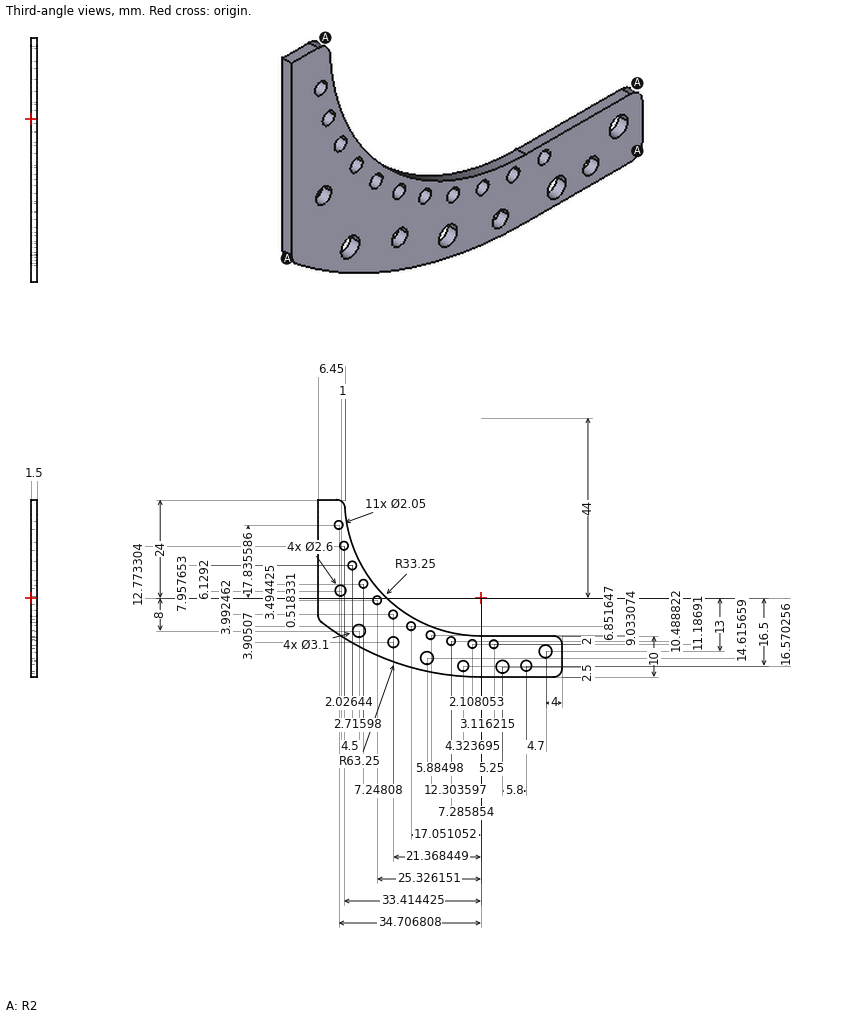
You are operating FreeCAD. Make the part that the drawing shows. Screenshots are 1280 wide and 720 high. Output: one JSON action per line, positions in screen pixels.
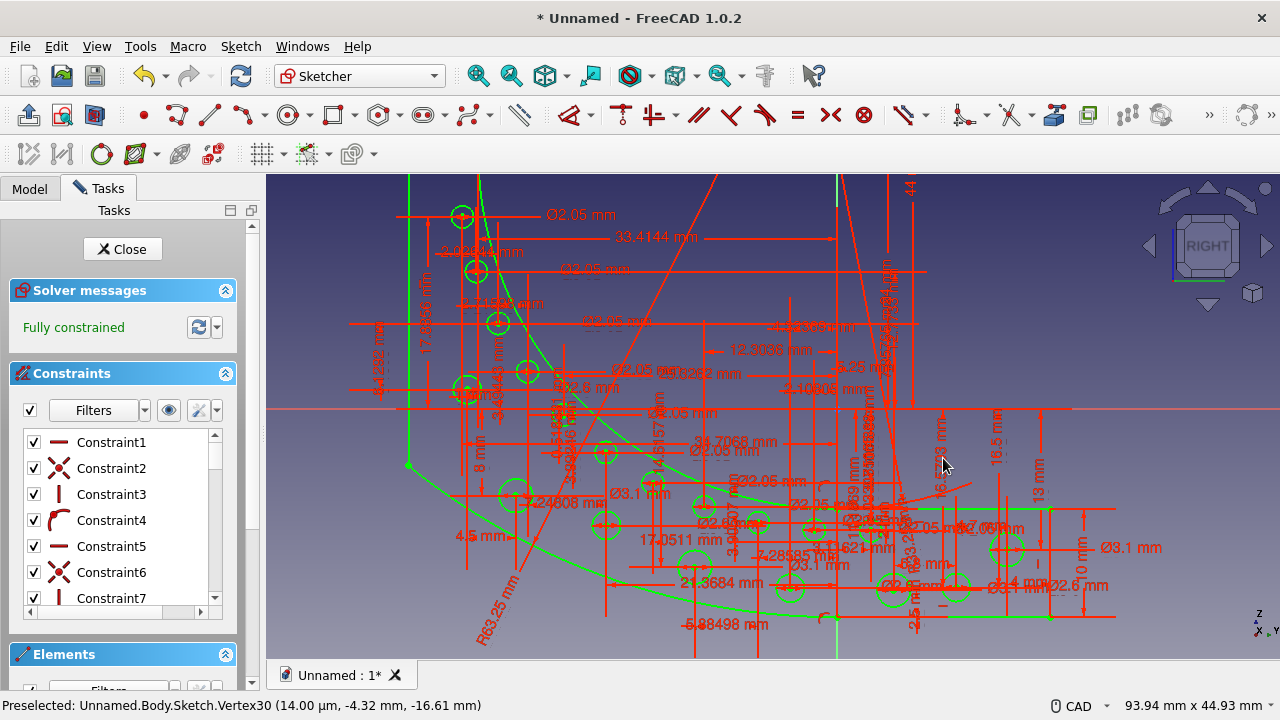
{"action": "left_click", "coordinate": [123, 249]}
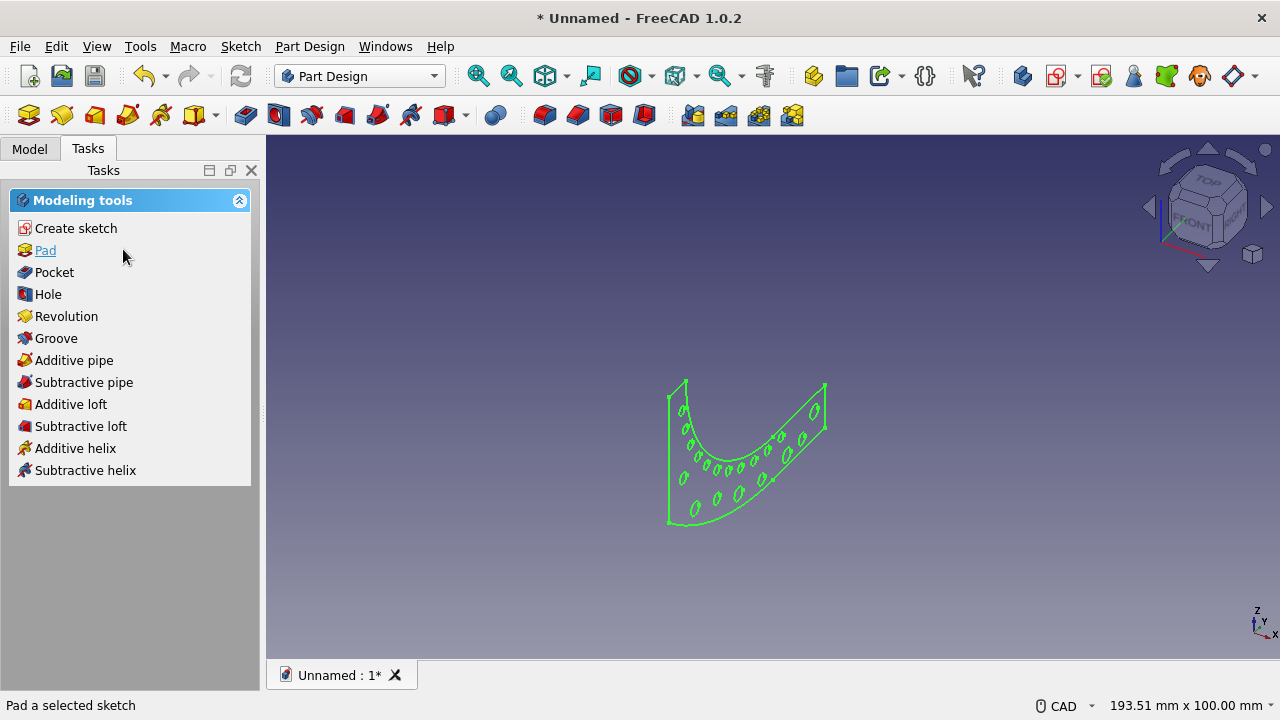
{"action": "left_click", "coordinate": [29, 116]}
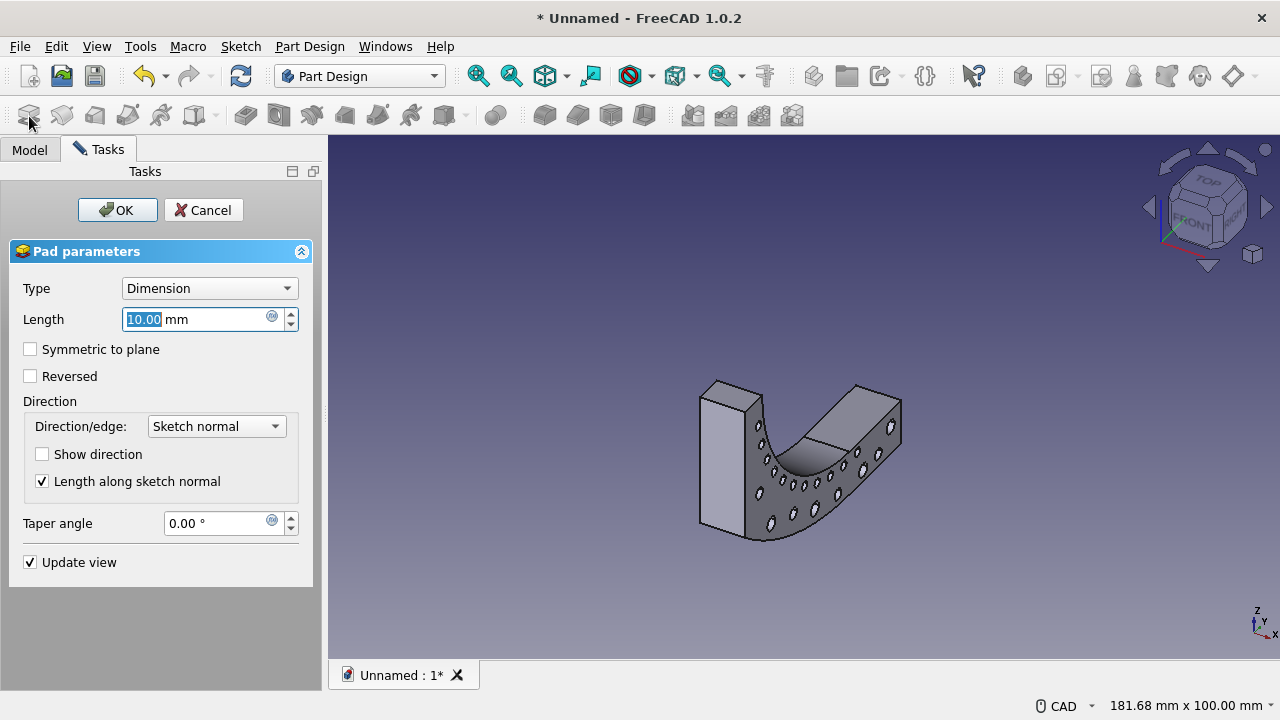
{"action": "type", "text": "1.5"}
{"action": "key", "text": "Tab"}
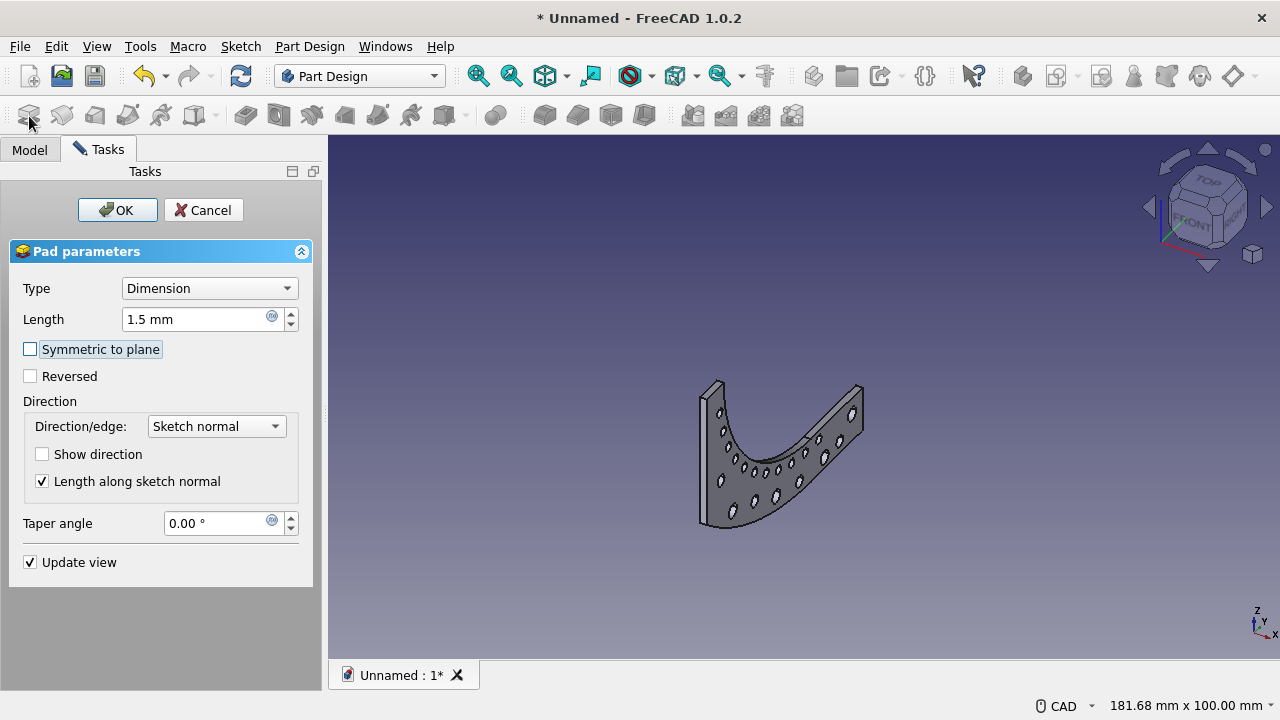
{"action": "left_click", "coordinate": [118, 210]}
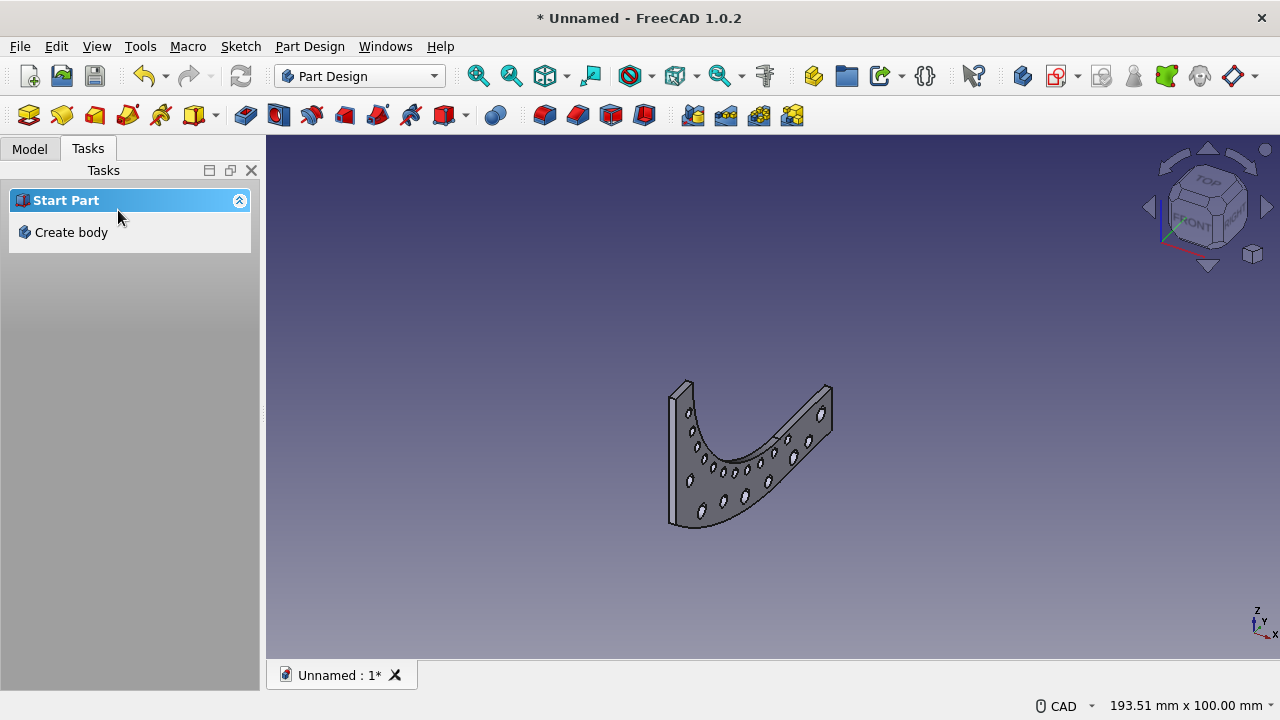
{"action": "scroll", "coordinate": [828, 428], "scroll_direction": "up", "scroll_amount": 9}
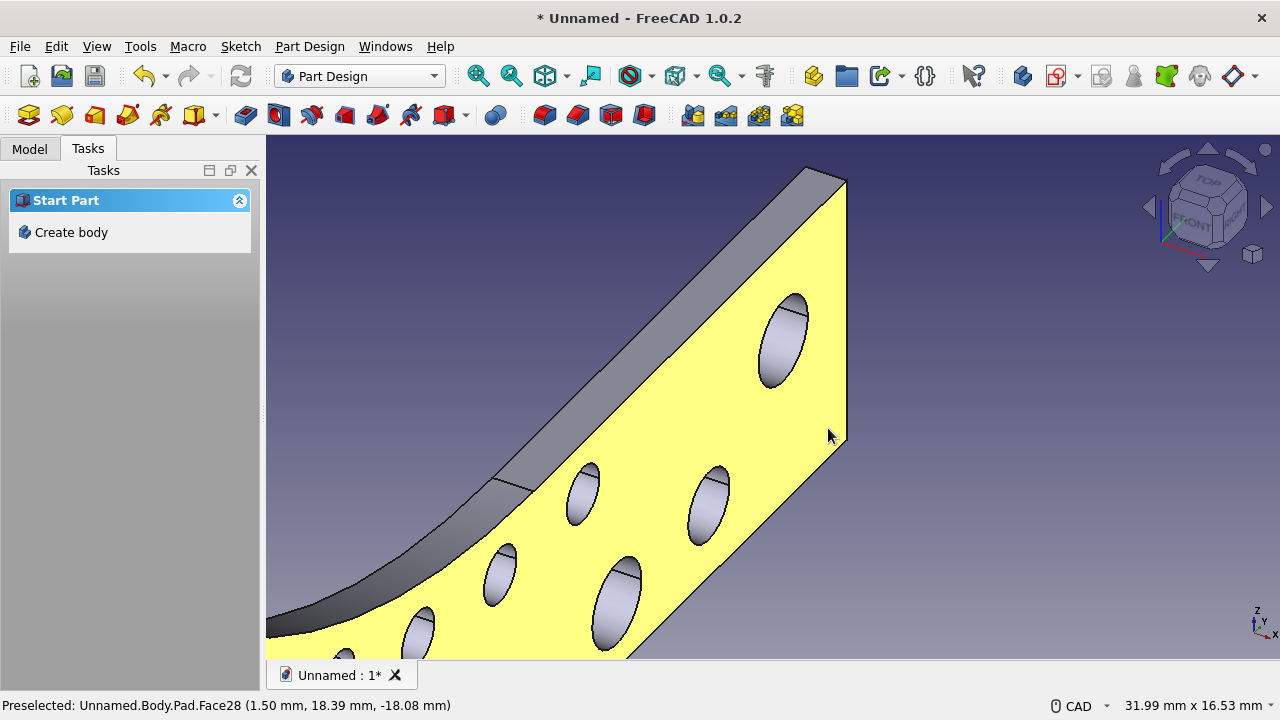
{"action": "left_click", "coordinate": [479, 76]}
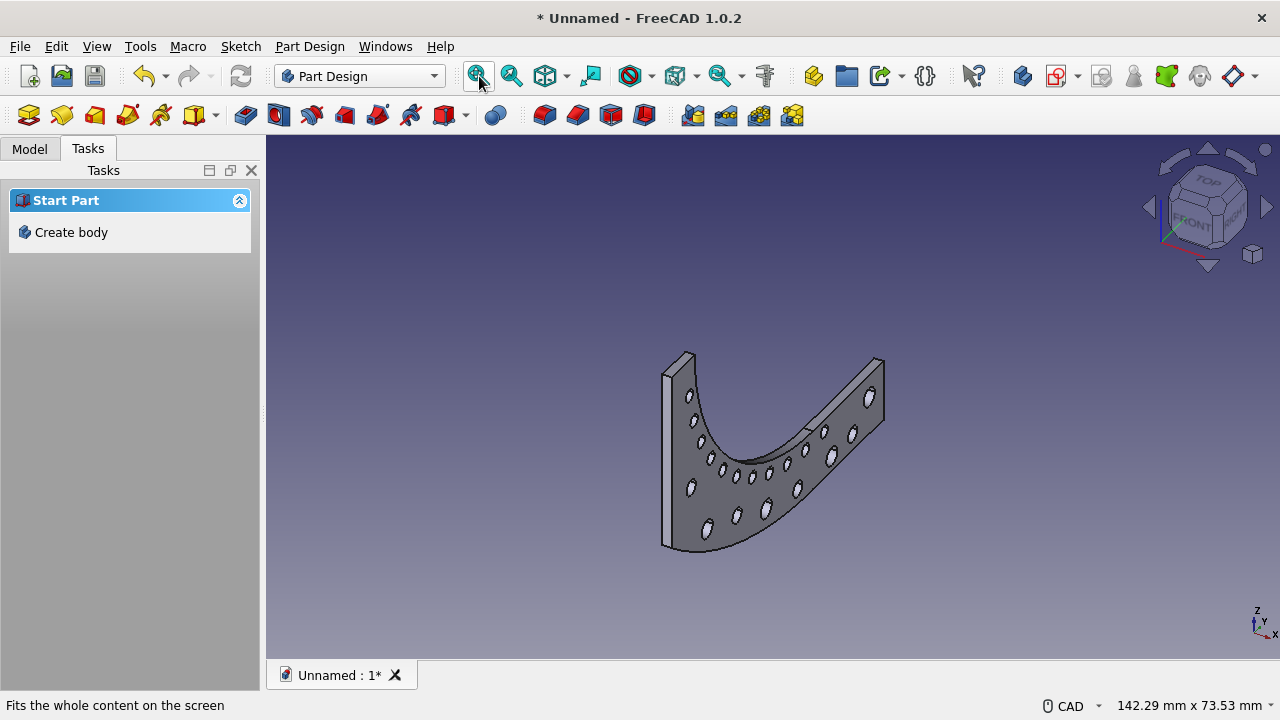
{"action": "key", "text": "0"}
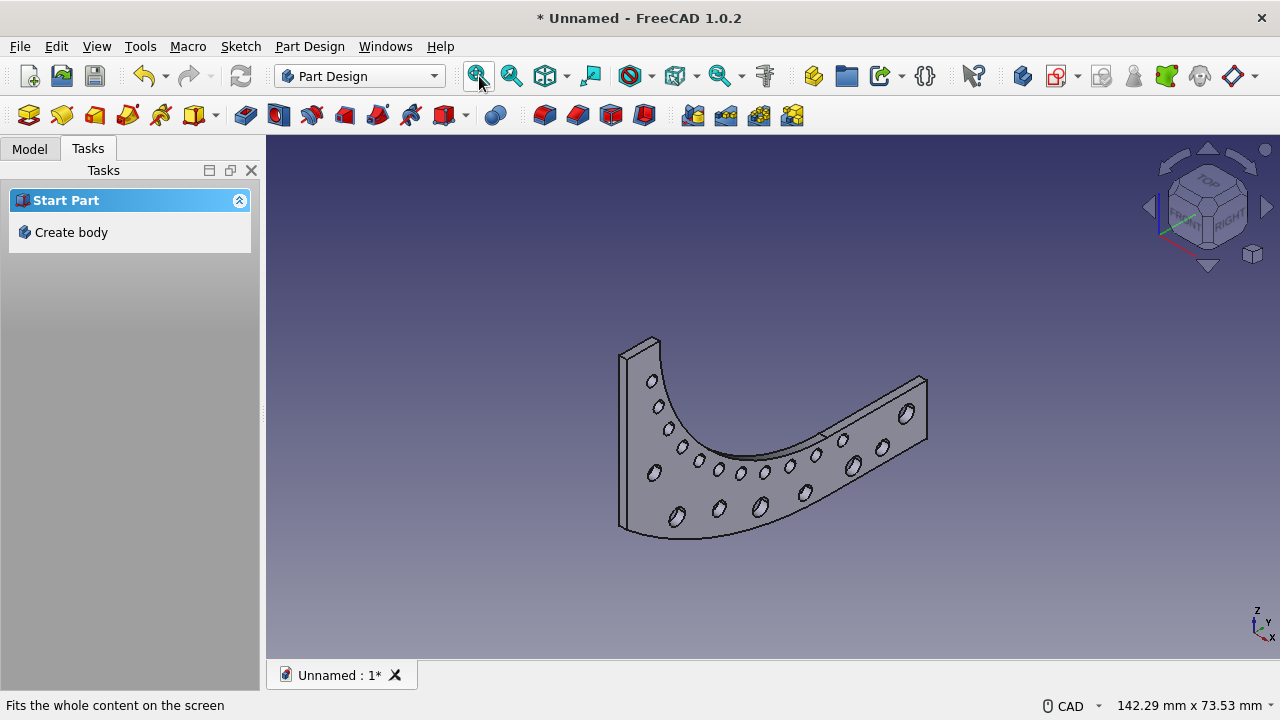
{"action": "scroll", "coordinate": [923, 435], "scroll_direction": "up", "scroll_amount": 7}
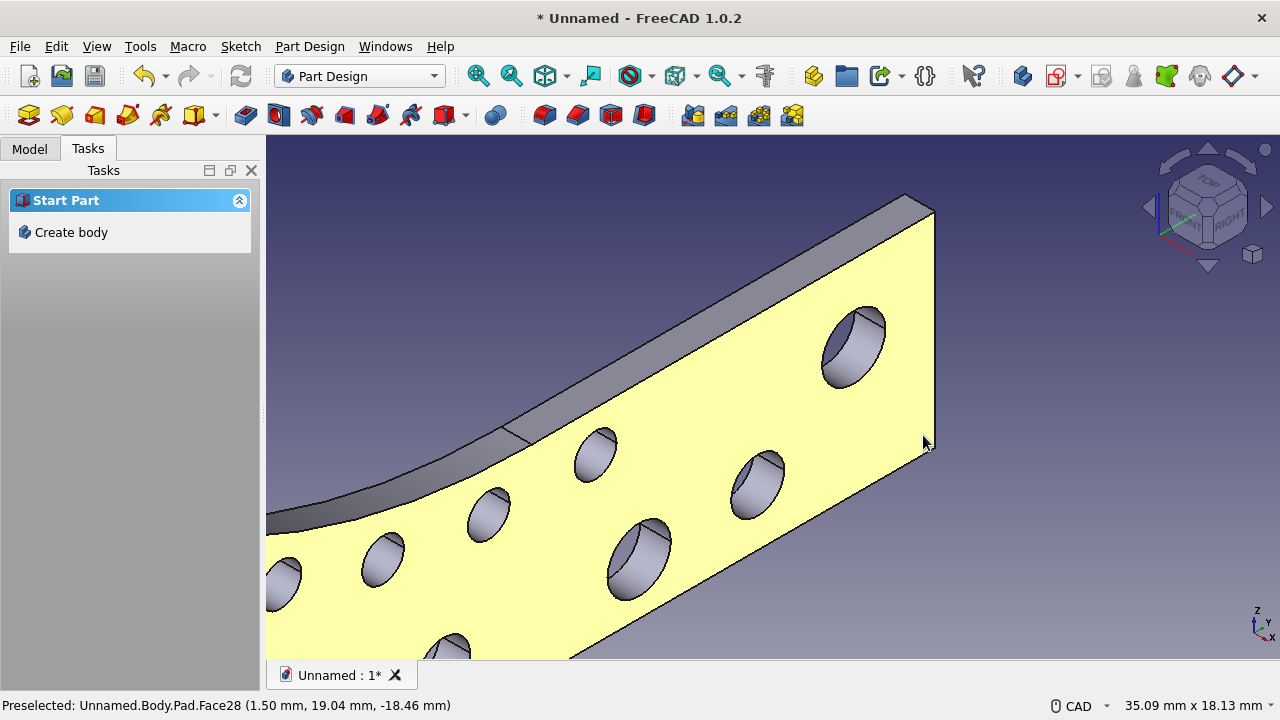
{"action": "key", "text": "v f"}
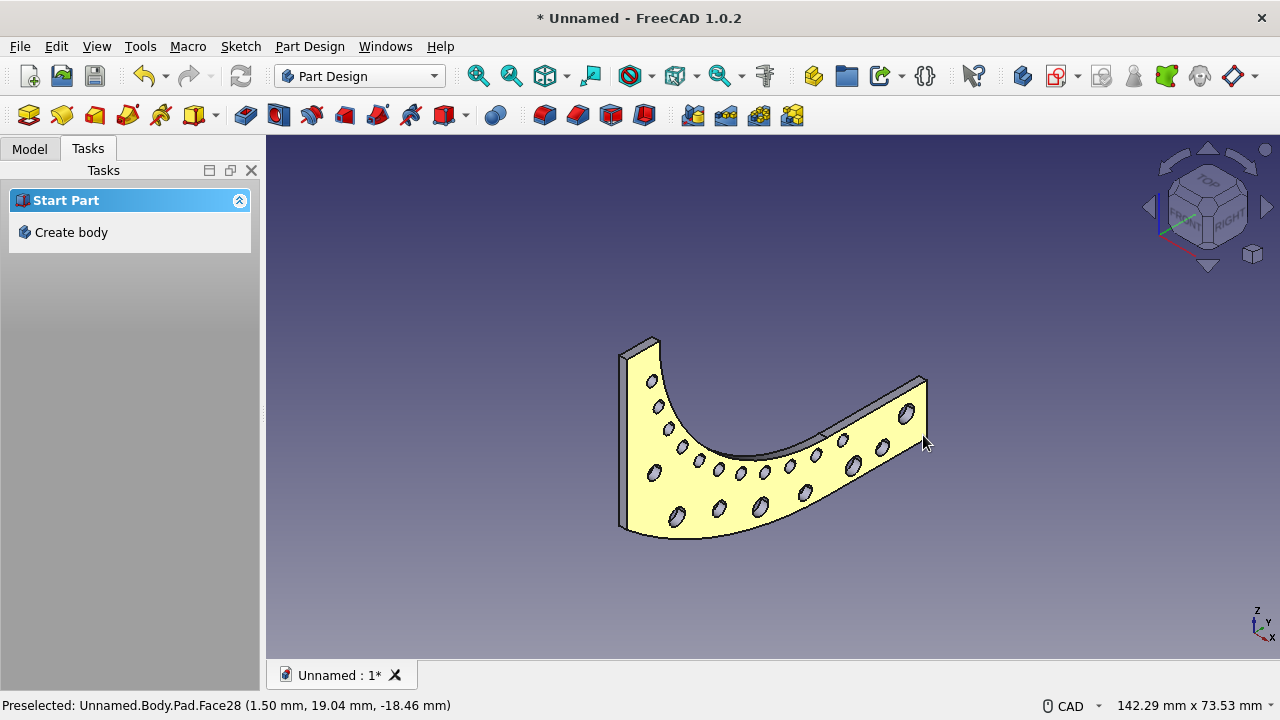
{"action": "key", "text": "2"}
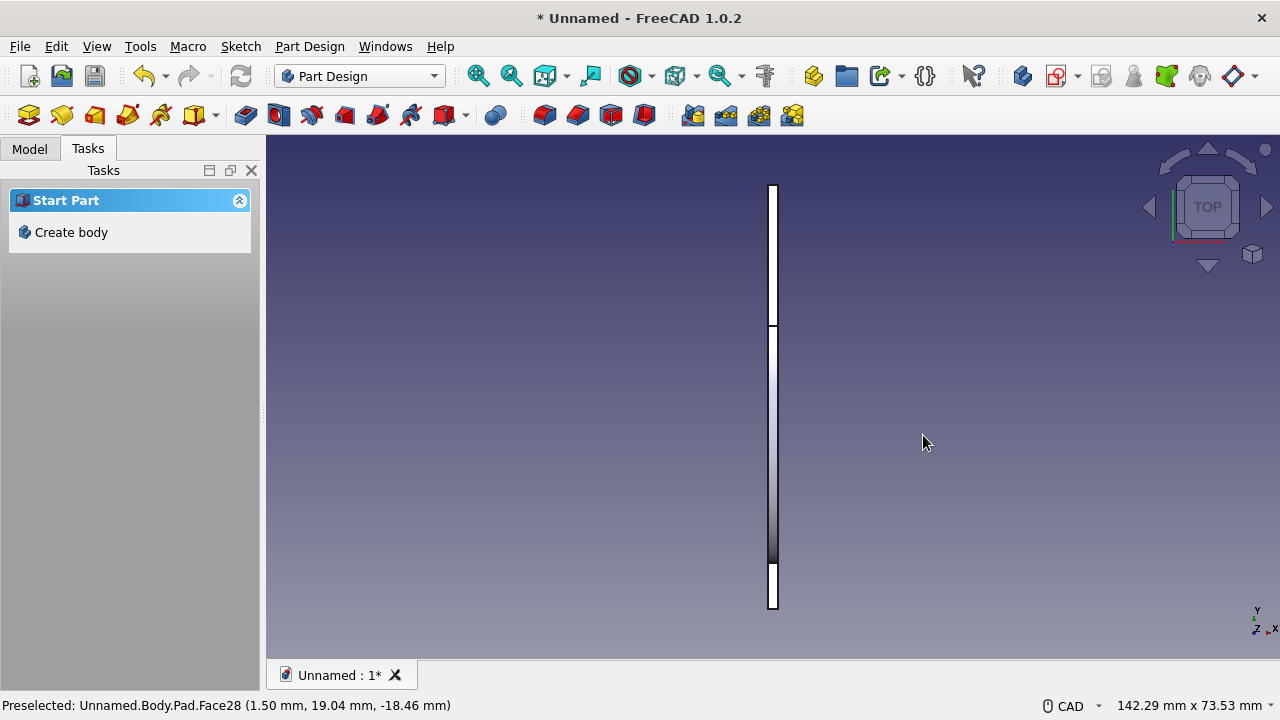
{"action": "scroll", "coordinate": [773, 184], "scroll_direction": "up", "scroll_amount": 7}